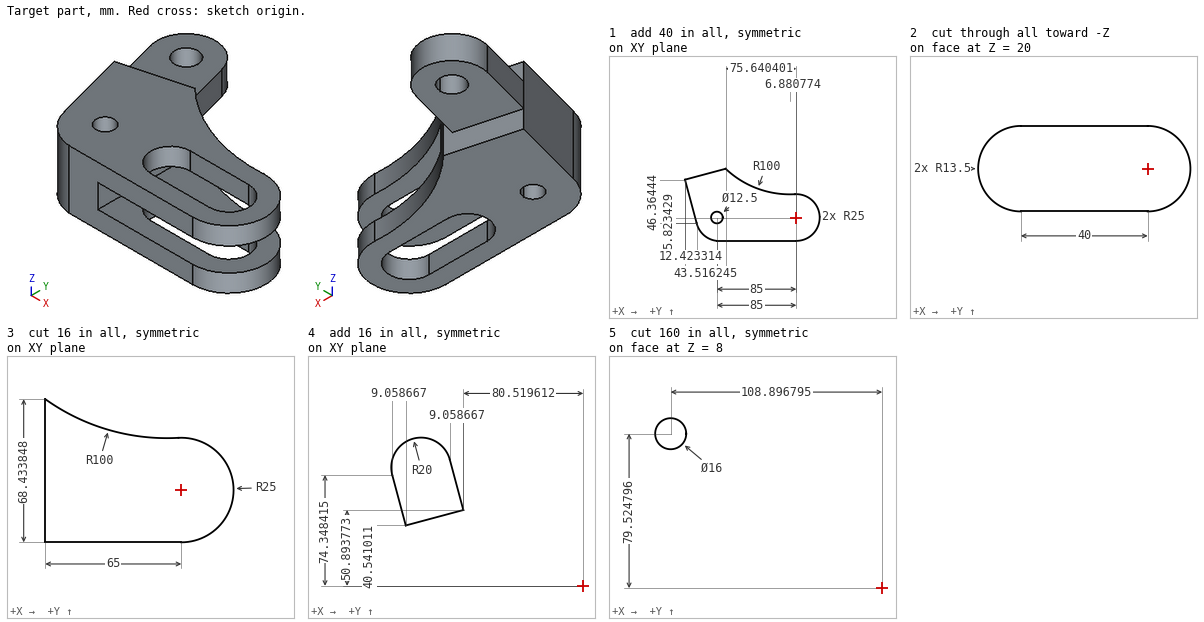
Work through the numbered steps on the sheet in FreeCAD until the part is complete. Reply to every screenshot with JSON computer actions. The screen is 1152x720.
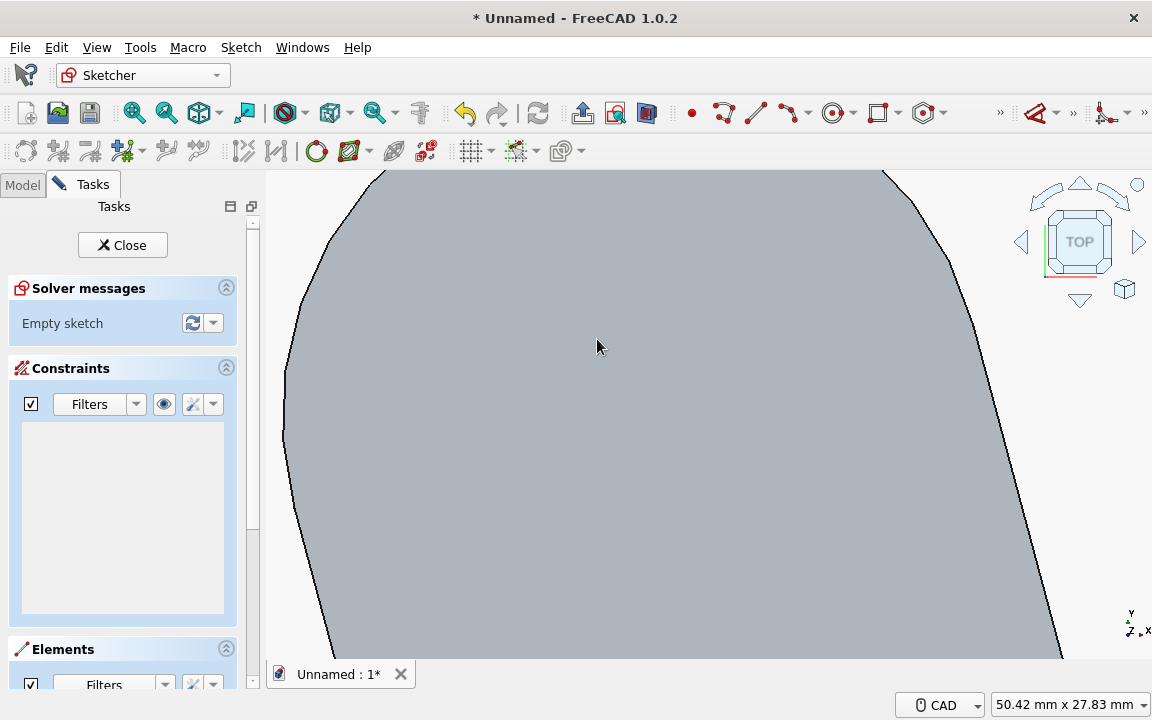
{"action": "left_click", "coordinate": [834, 114]}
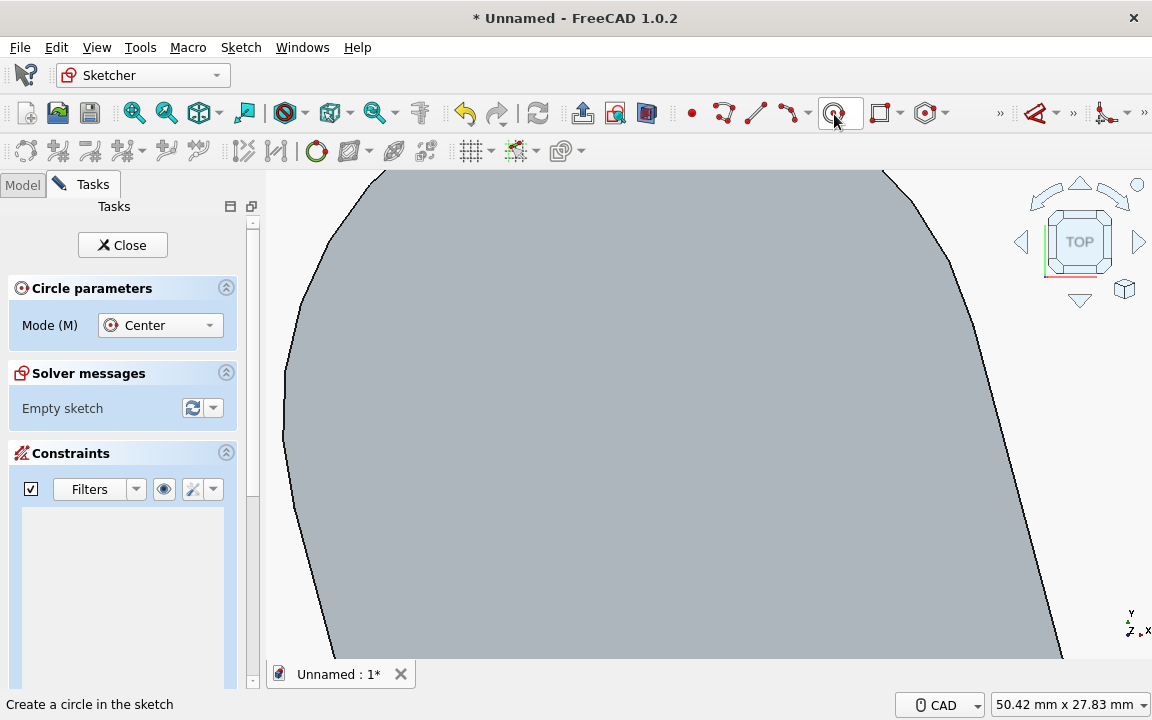
{"action": "left_click", "coordinate": [634, 417]}
{"action": "mouse_move", "coordinate": [733, 317]}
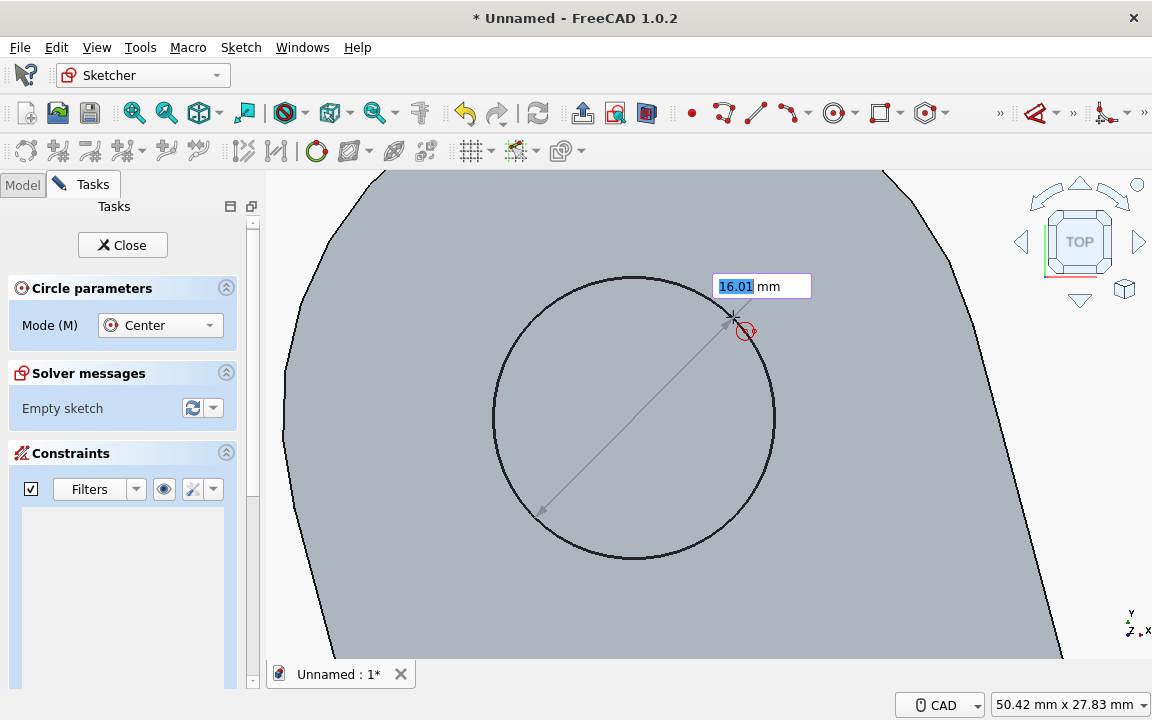
{"action": "type", "text": "16"}
{"action": "key", "text": "Return"}
{"action": "key", "text": "Escape"}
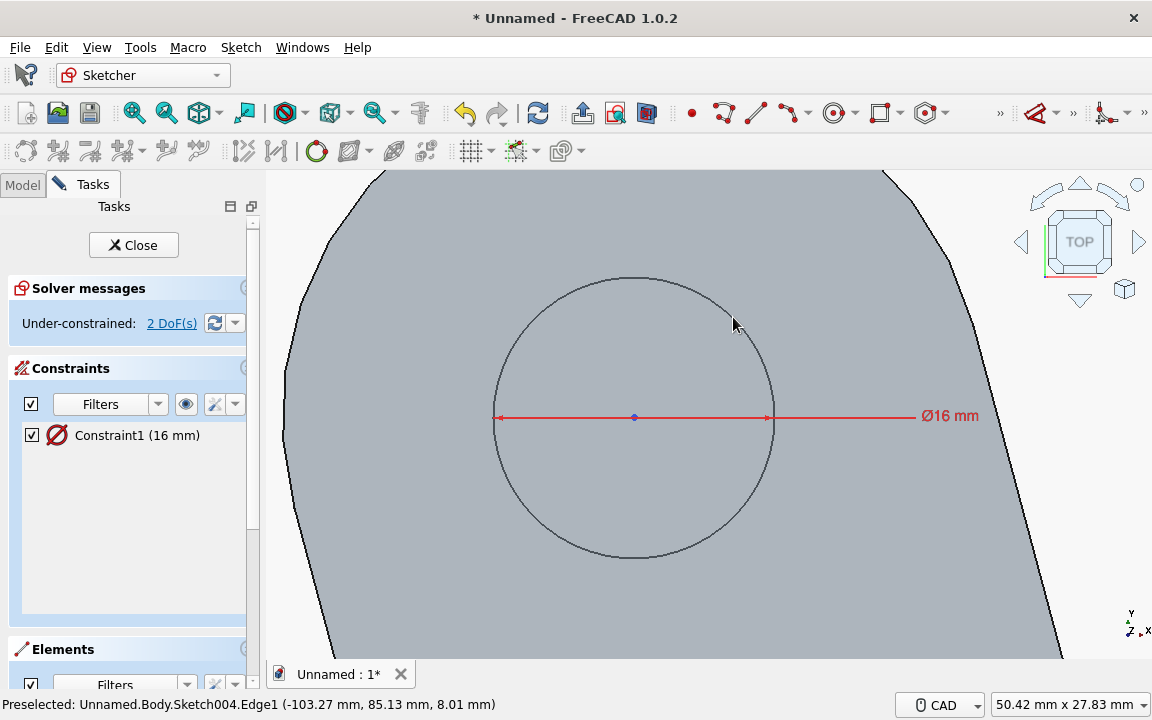
{"action": "left_click", "coordinate": [1036, 114]}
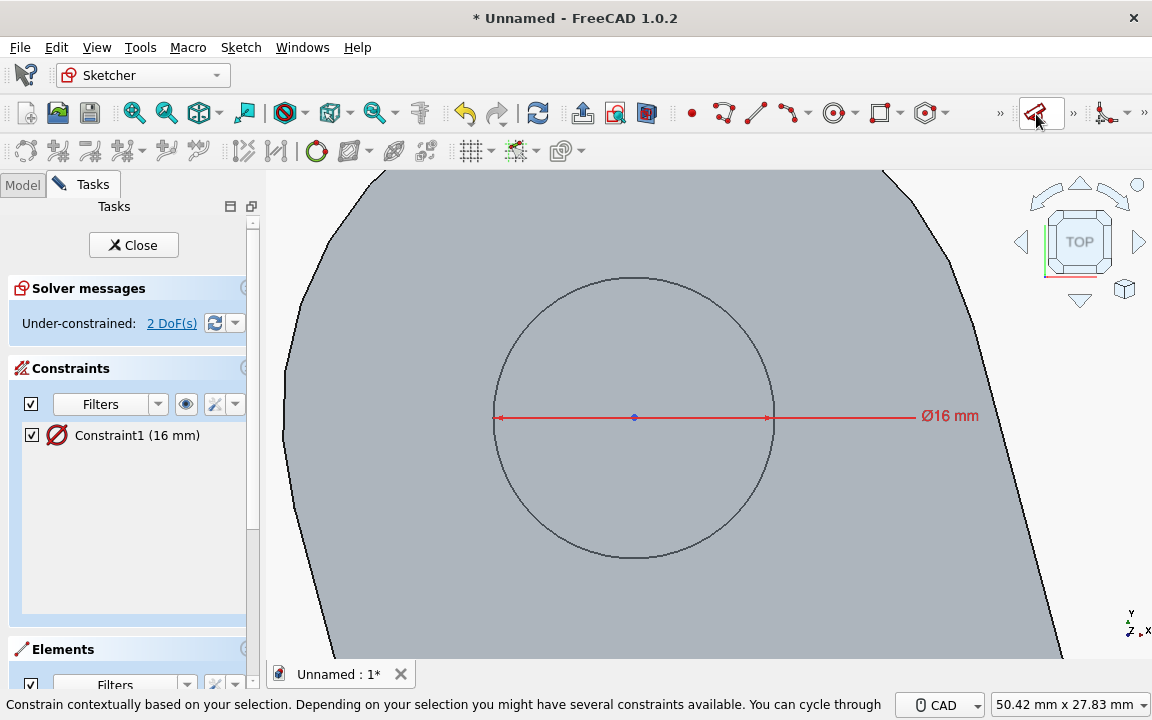
{"action": "left_click", "coordinate": [634, 418]}
{"action": "left_click", "coordinate": [600, 524]}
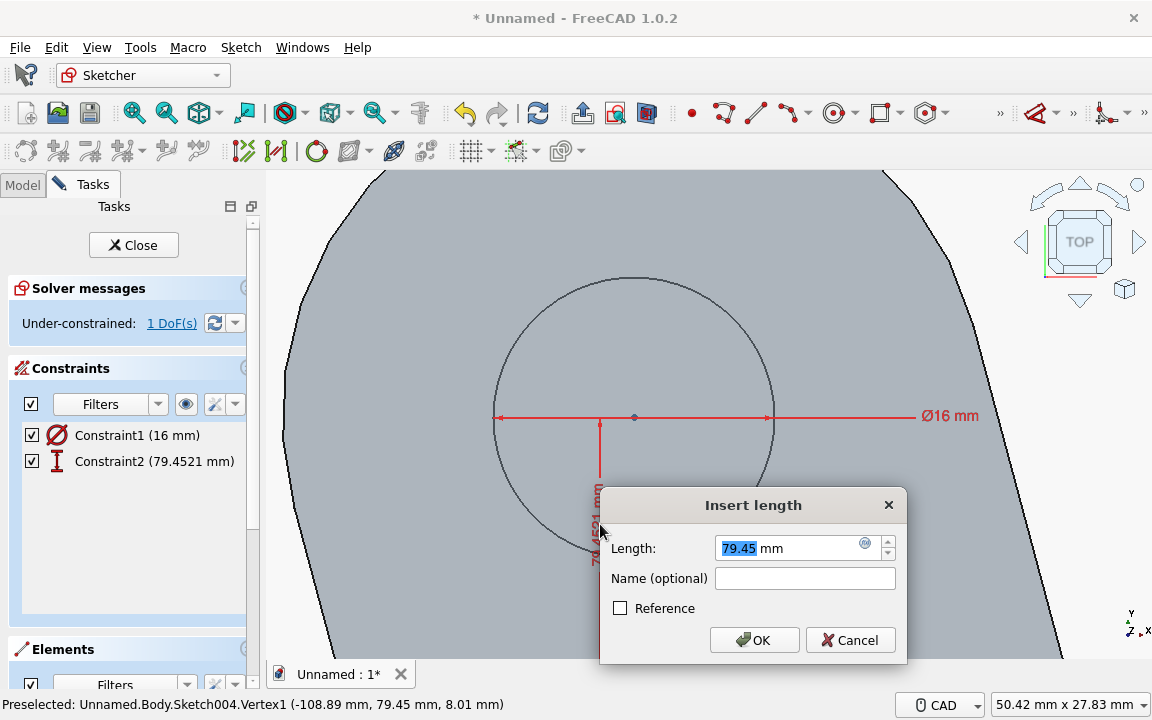
{"action": "type", "text": "79.524796"}
{"action": "key", "text": "Return"}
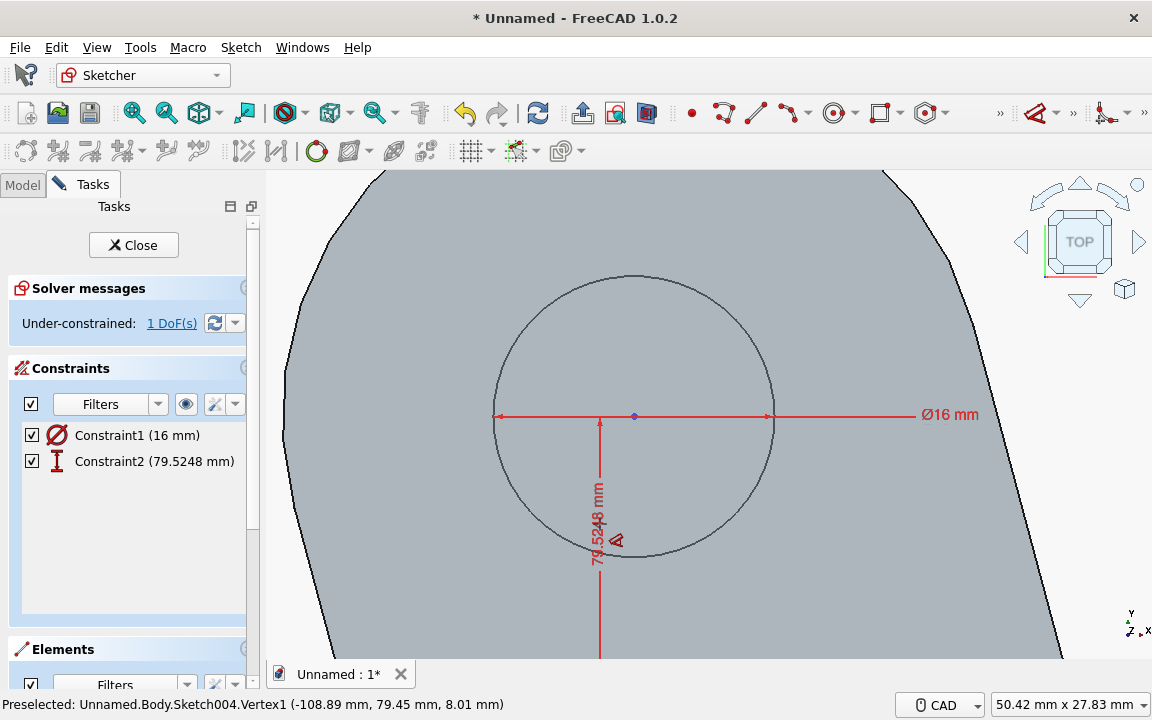
{"action": "left_click", "coordinate": [634, 417]}
{"action": "left_click", "coordinate": [811, 383]}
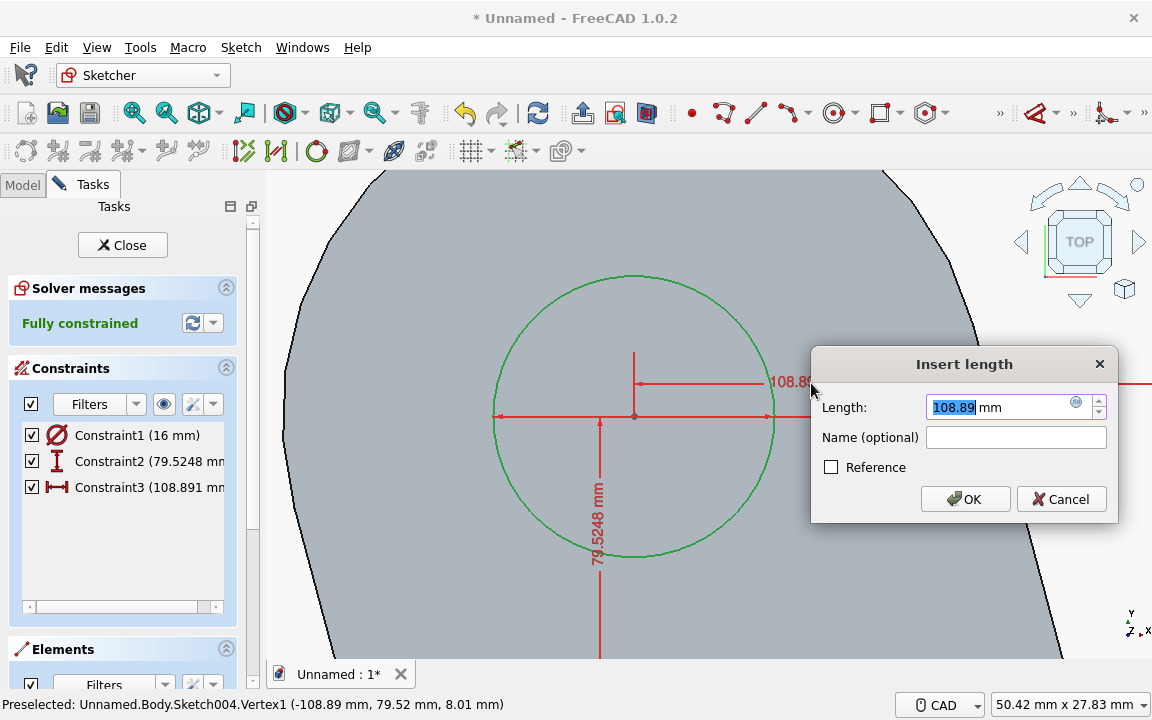
{"action": "type", "text": "108.896795"}
{"action": "key", "text": "Return"}
{"action": "key", "text": "Escape"}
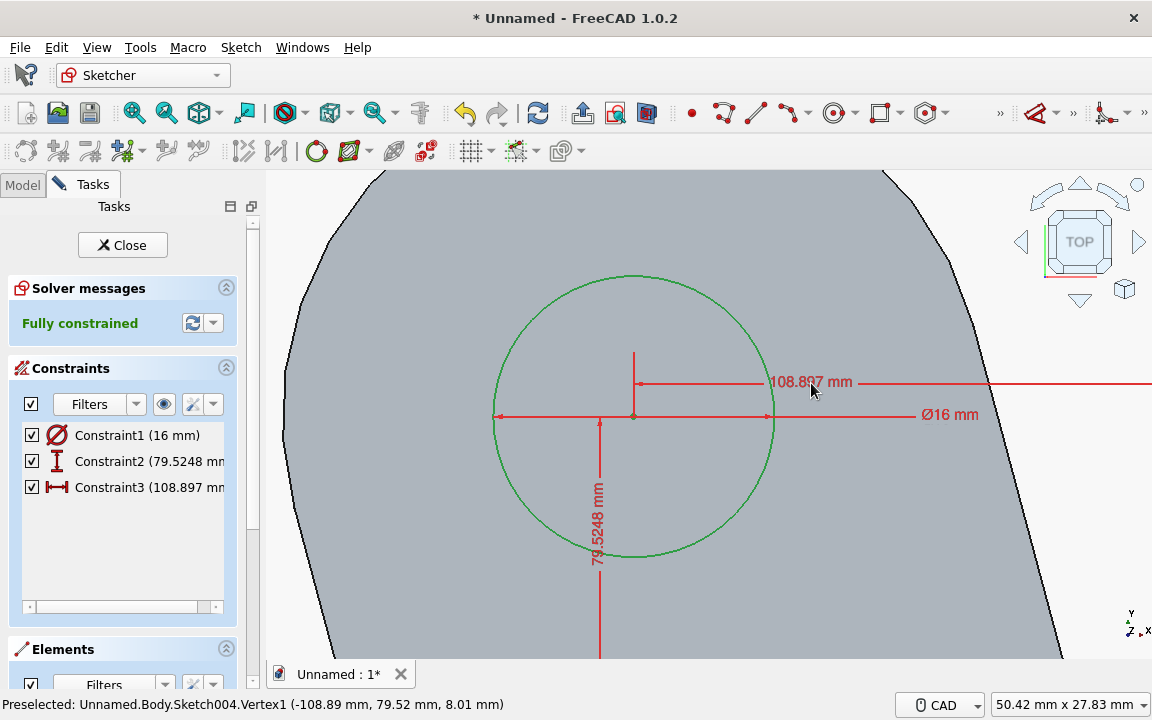
{"action": "left_click", "coordinate": [123, 245]}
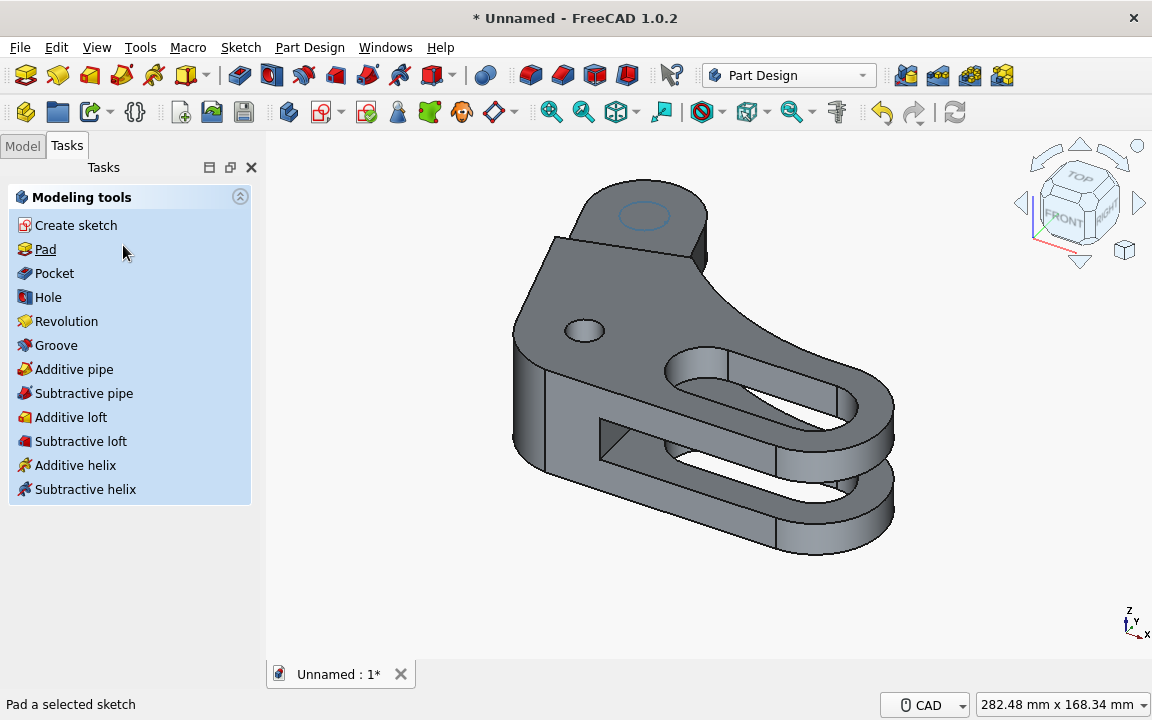
{"action": "left_click", "coordinate": [240, 76]}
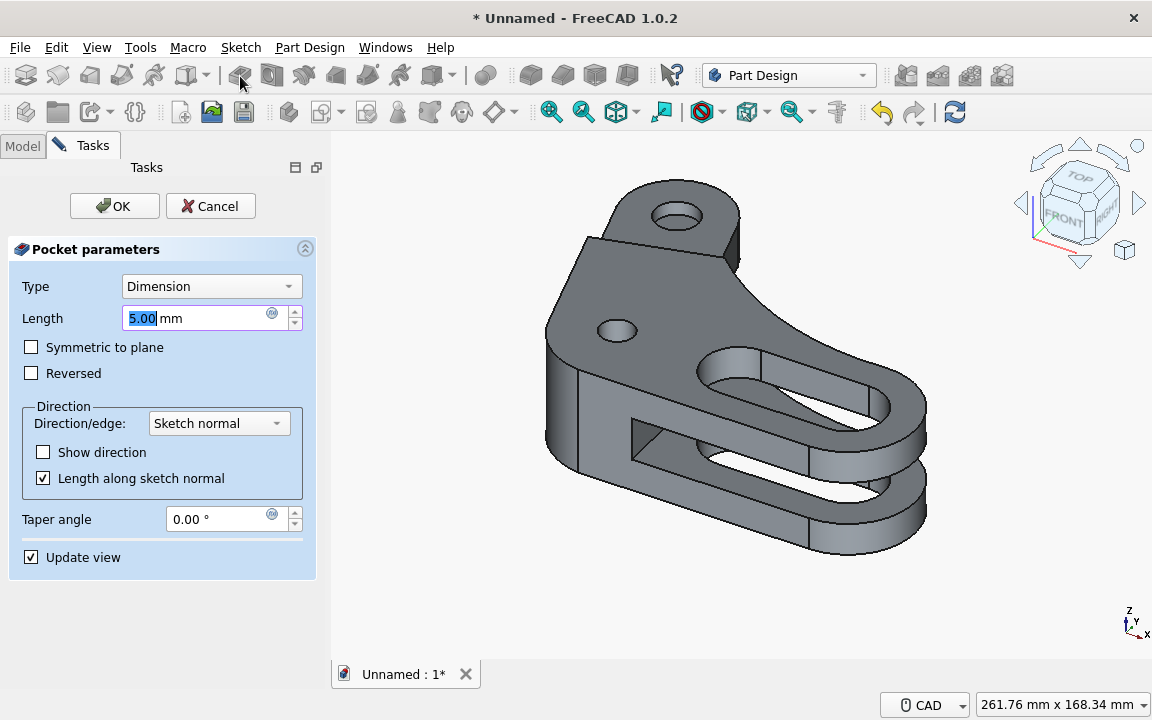
{"action": "type", "text": "160"}
{"action": "key", "text": "Tab"}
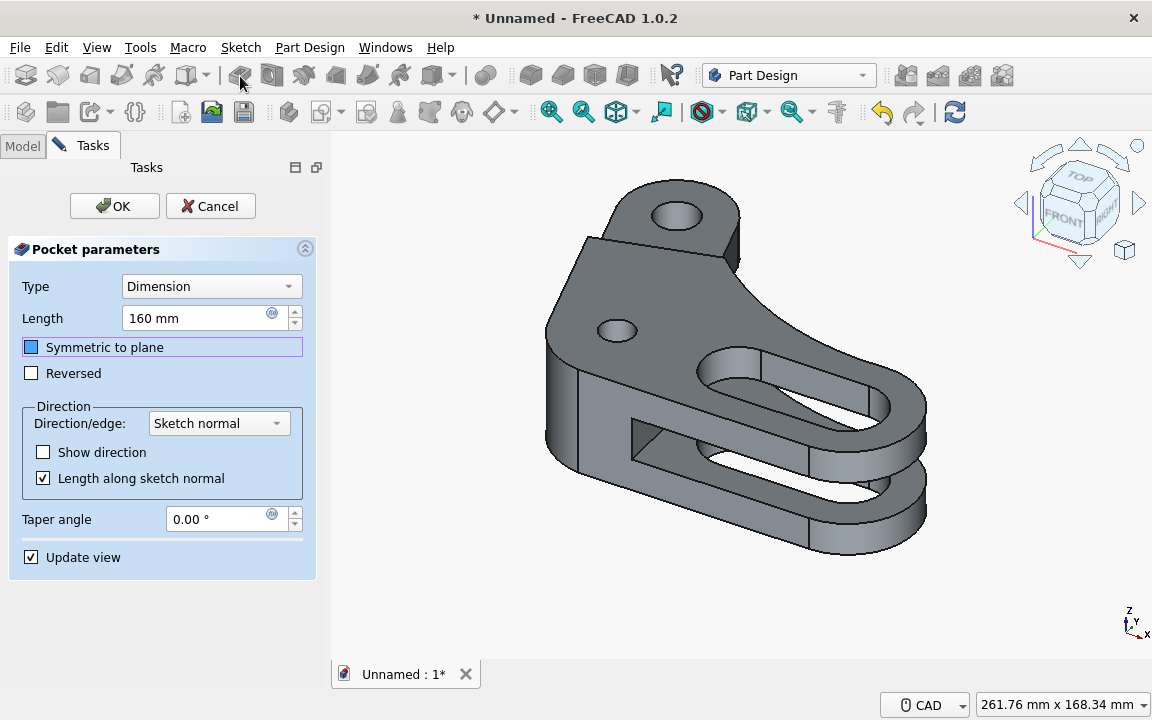
{"action": "left_click", "coordinate": [30, 347]}